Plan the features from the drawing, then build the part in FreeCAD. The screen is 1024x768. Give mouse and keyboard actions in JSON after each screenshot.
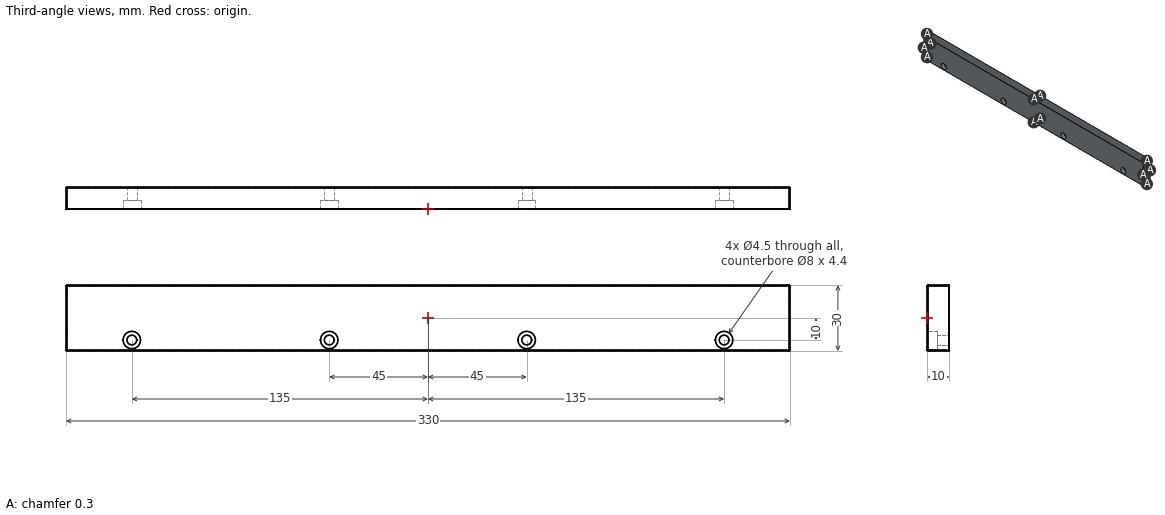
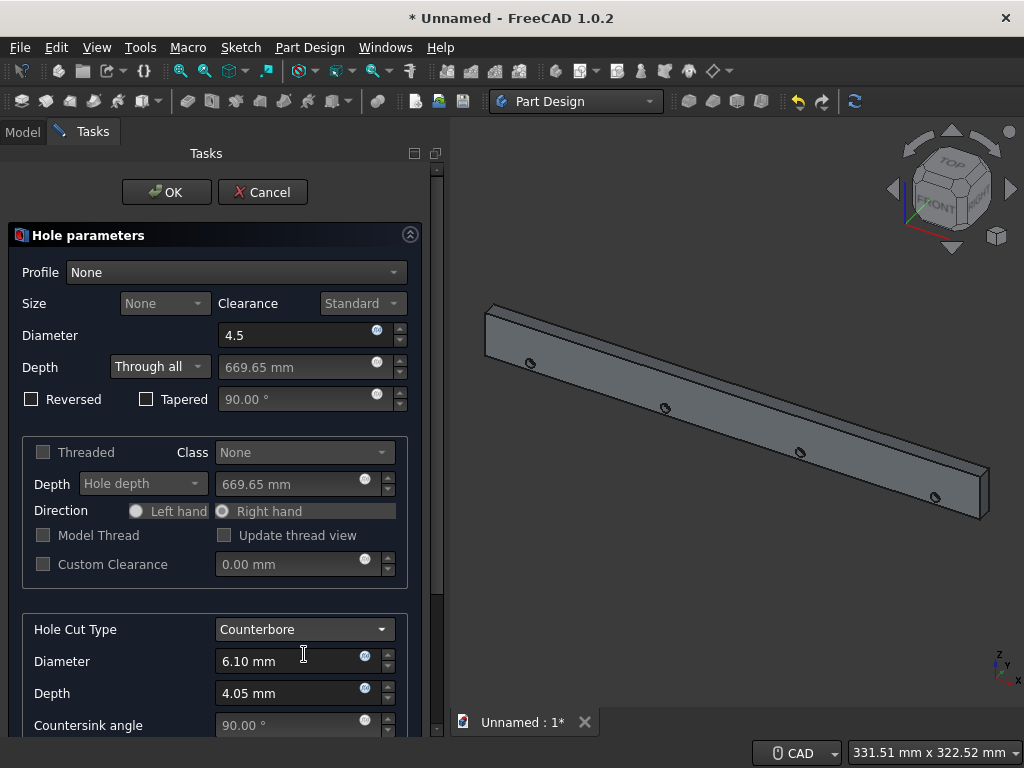
{"action": "triple_click", "coordinate": [298, 661]}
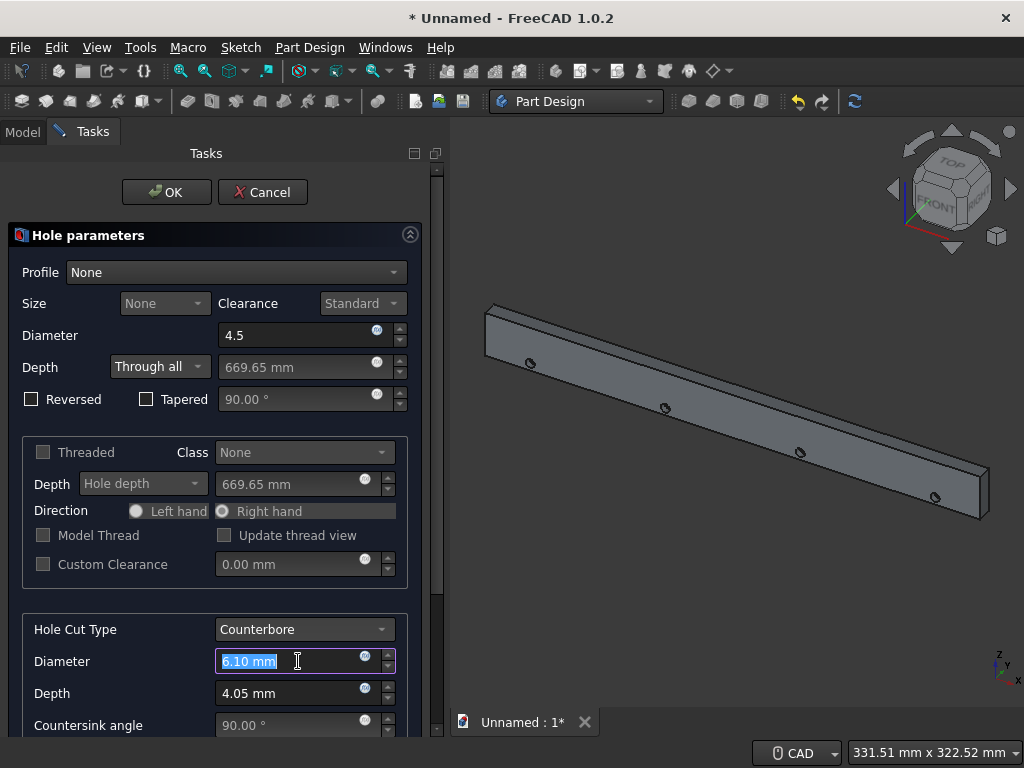
{"action": "type", "text": "8"}
{"action": "key", "text": "Tab"}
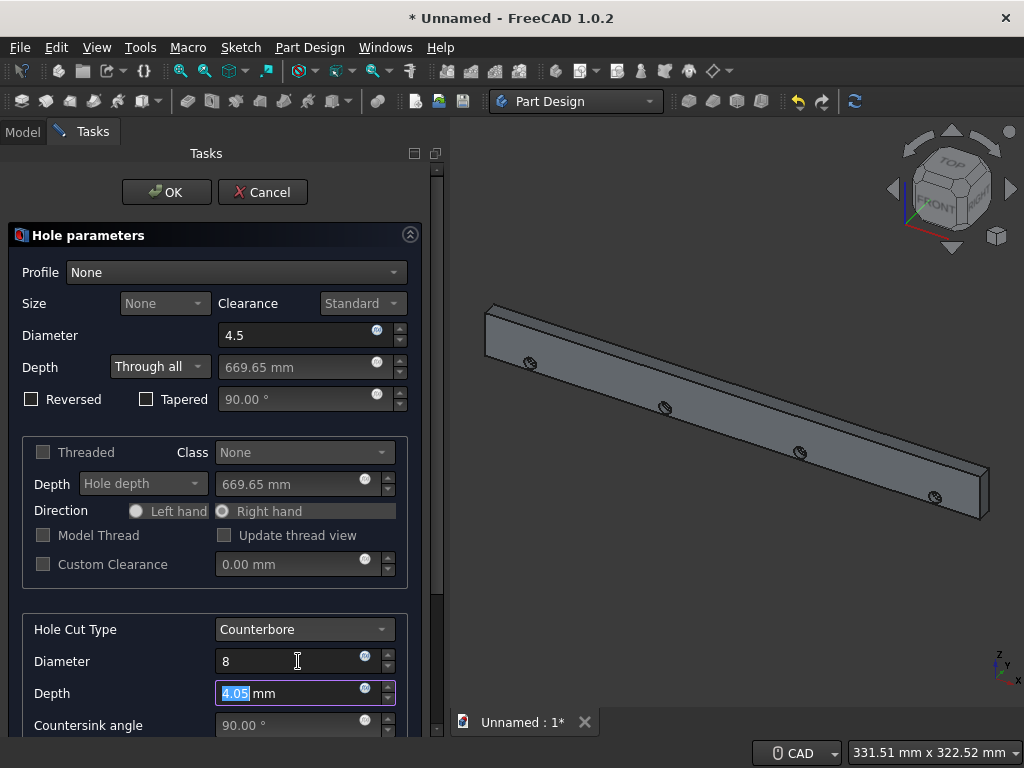
{"action": "type", "text": "4.4"}
{"action": "key", "text": "Tab"}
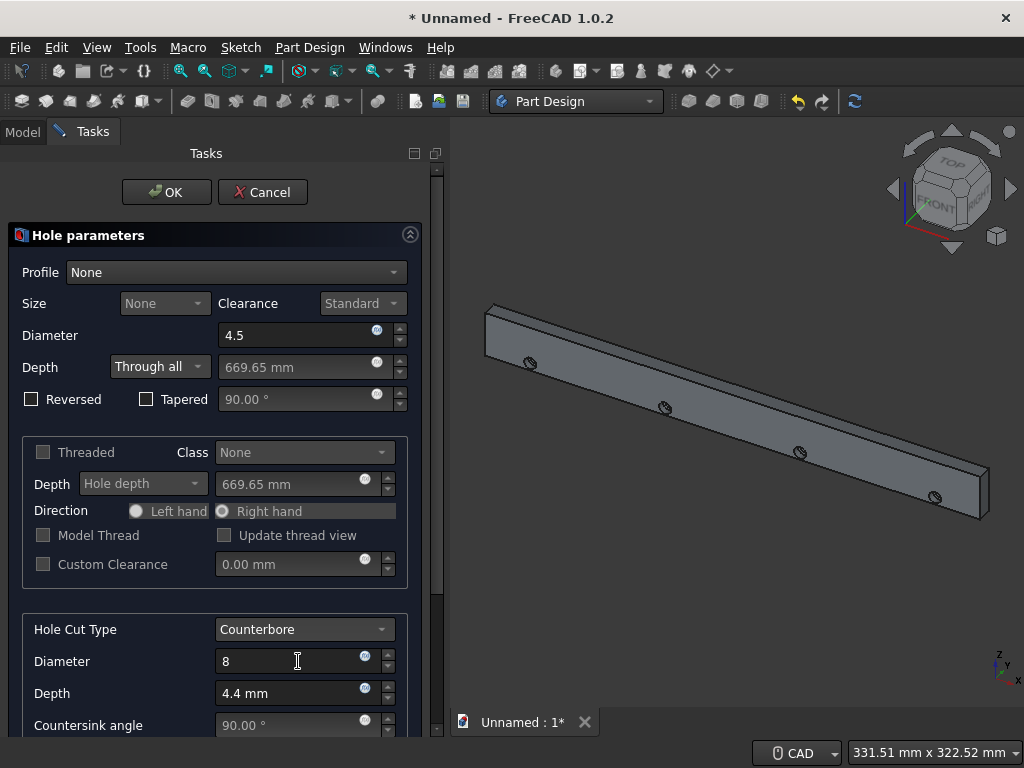
{"action": "left_click", "coordinate": [167, 192]}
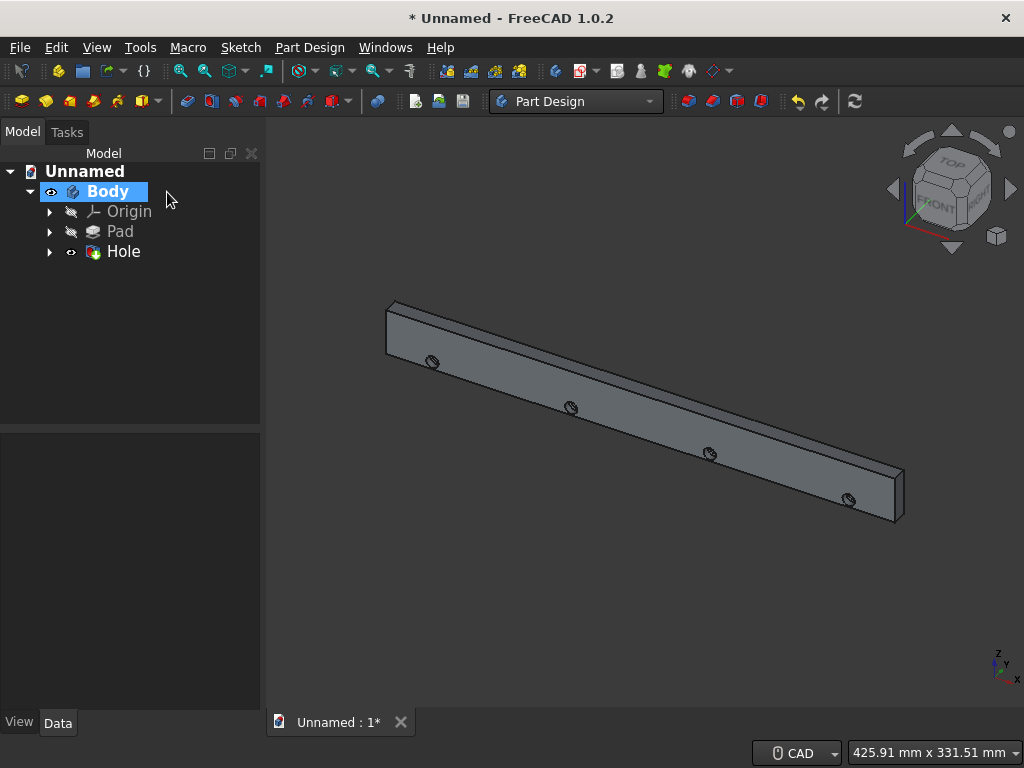
{"action": "left_click", "coordinate": [895, 500]}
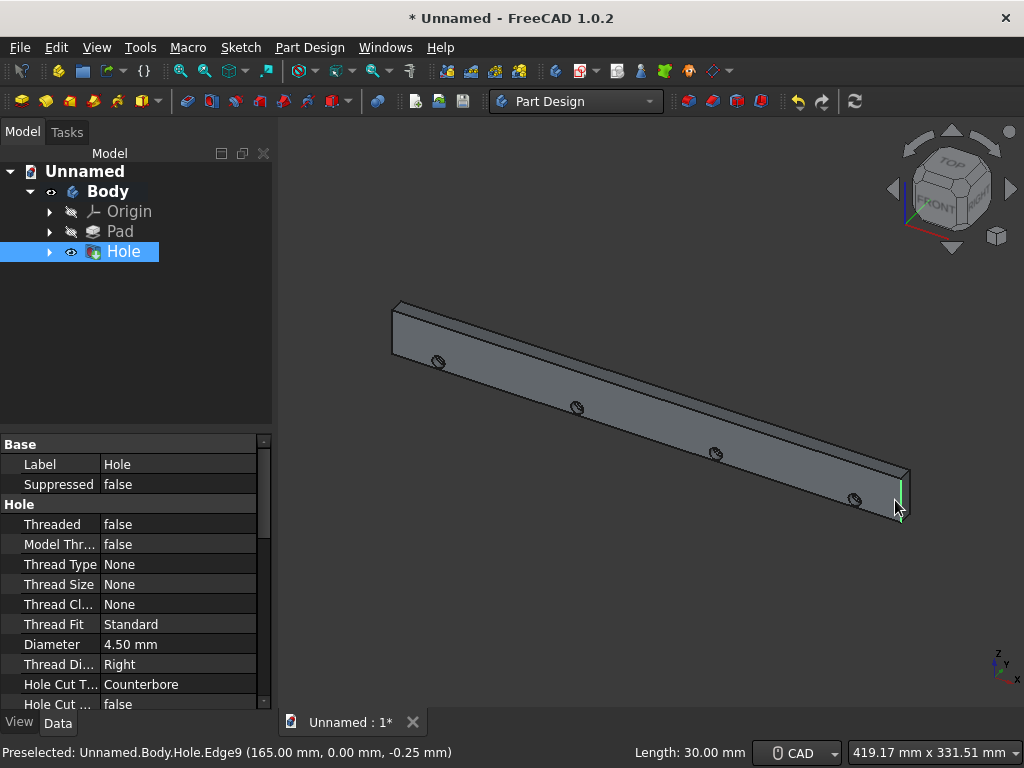
{"action": "key", "text": "0"}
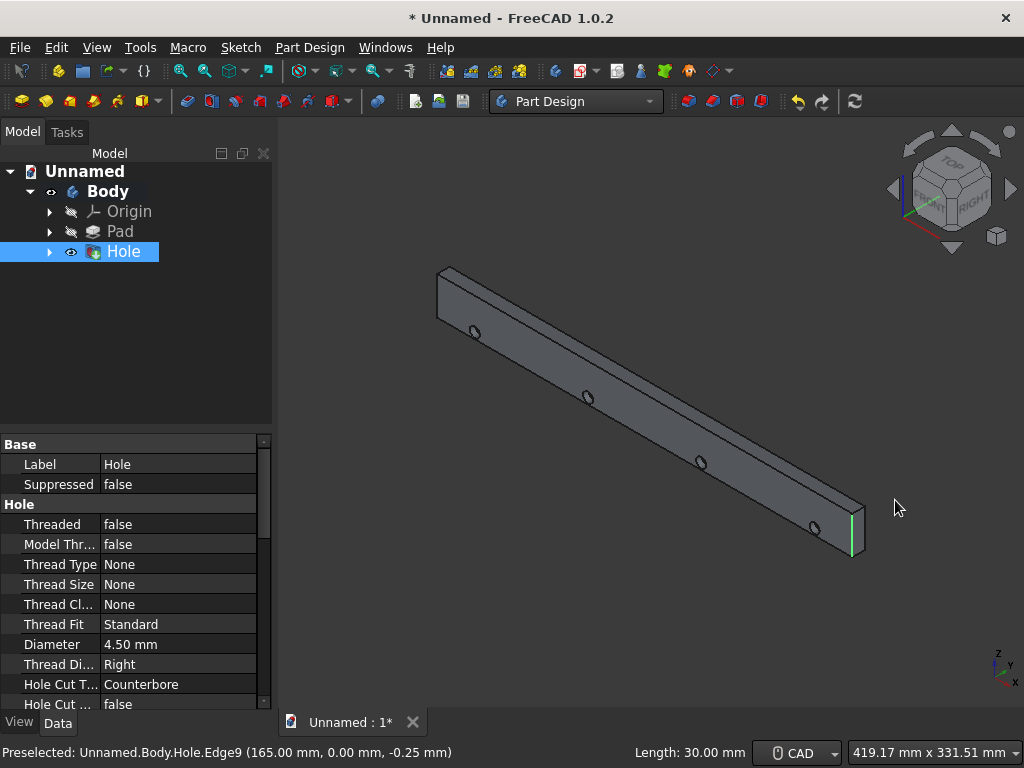
{"action": "key", "text": "2"}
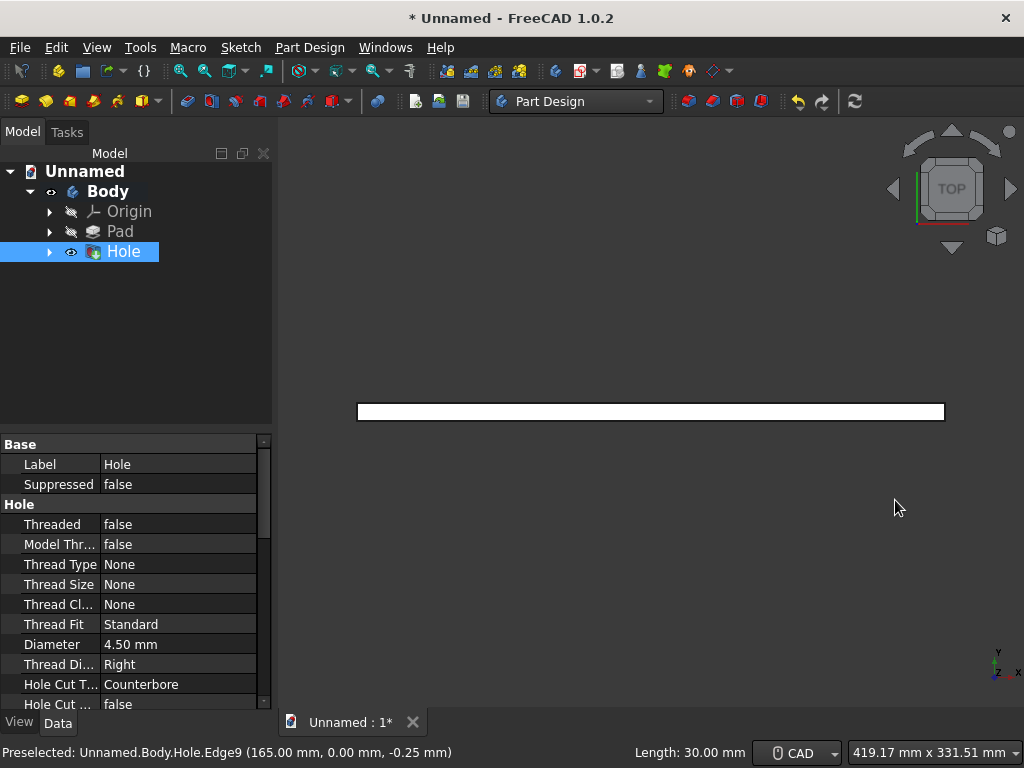
{"action": "left_click", "coordinate": [903, 411], "text": "ctrl"}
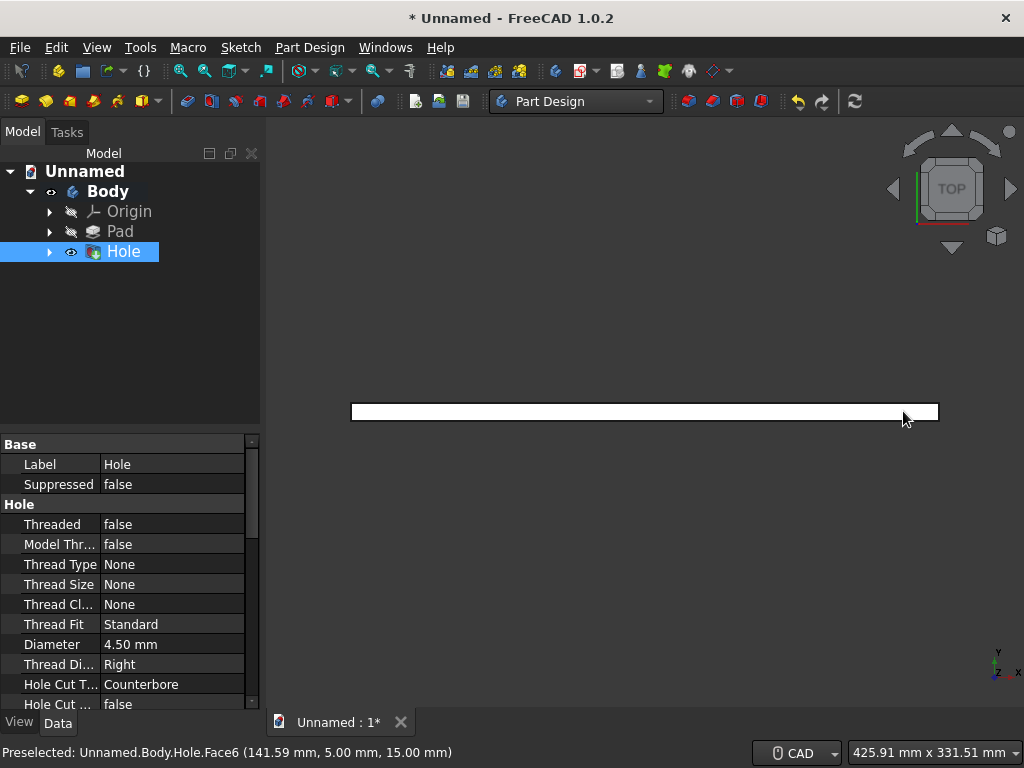
{"action": "key", "text": "1"}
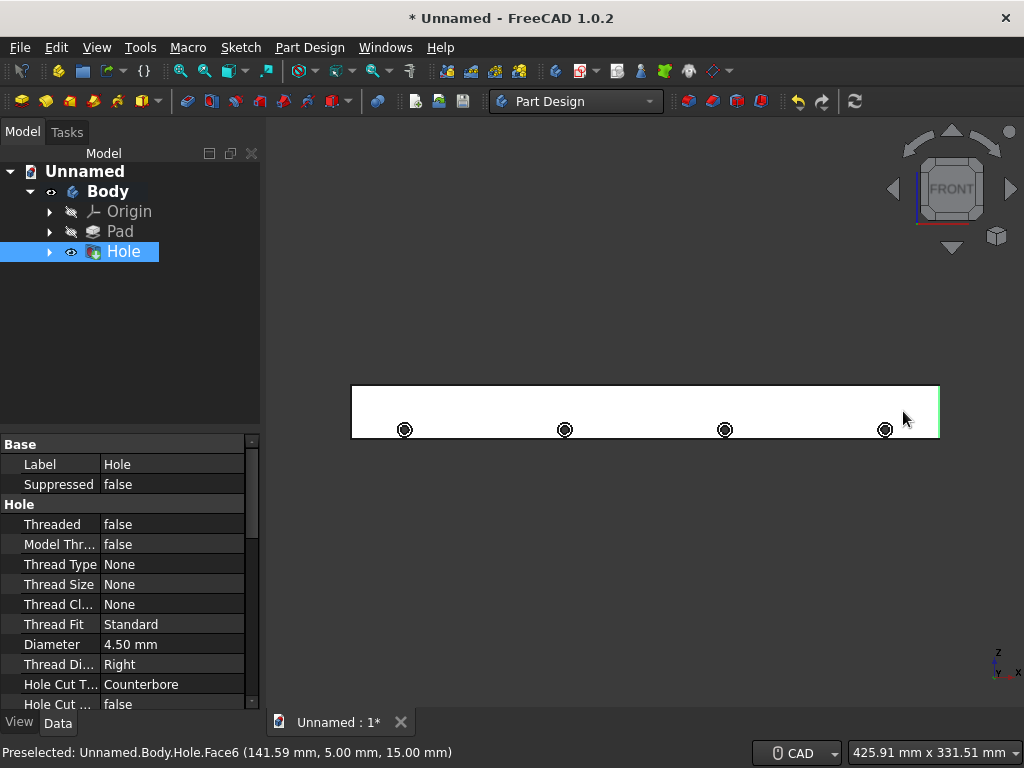
{"action": "left_click", "coordinate": [351, 411], "text": "ctrl"}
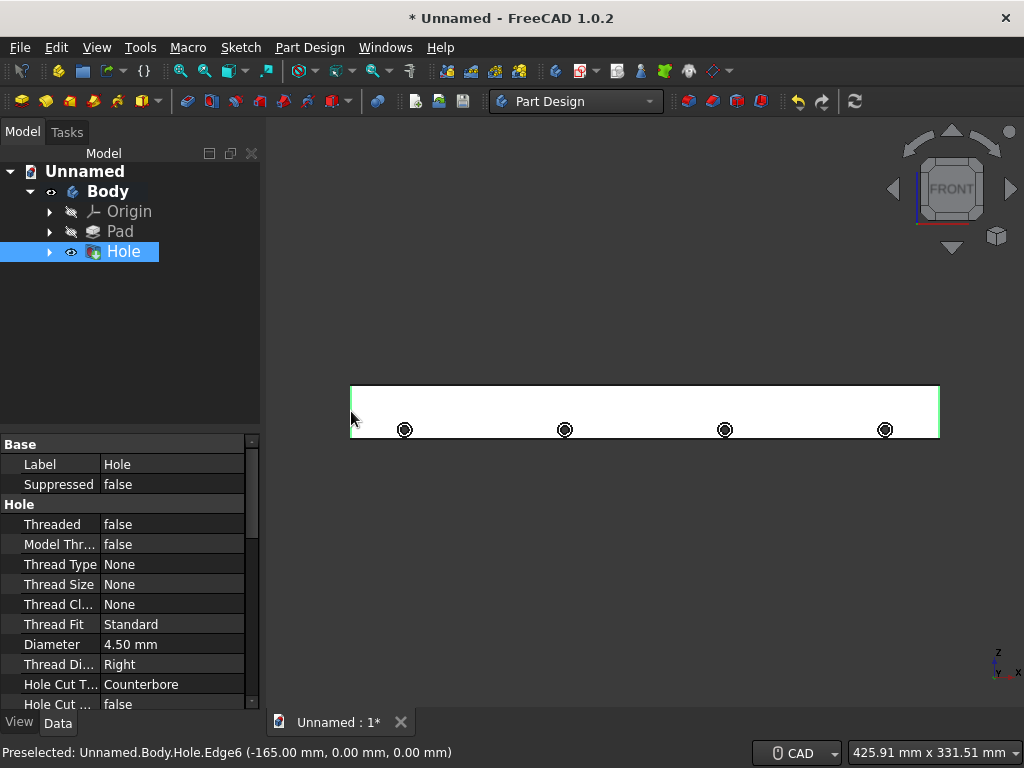
{"action": "key", "text": "3"}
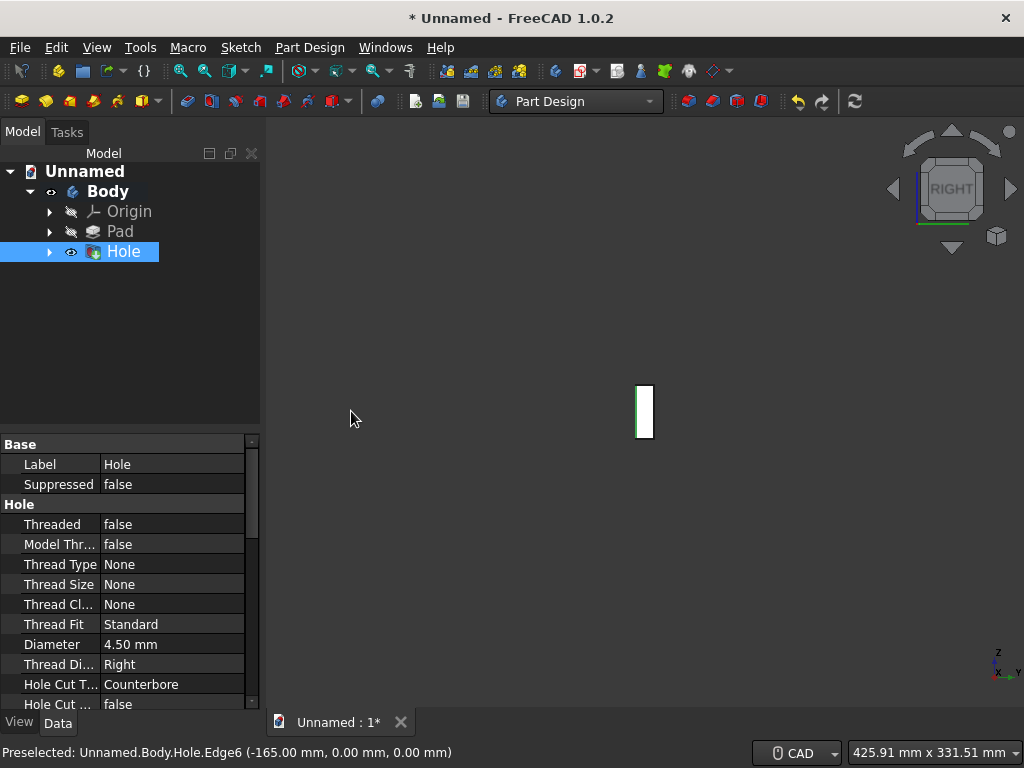
{"action": "left_click", "coordinate": [182, 72]}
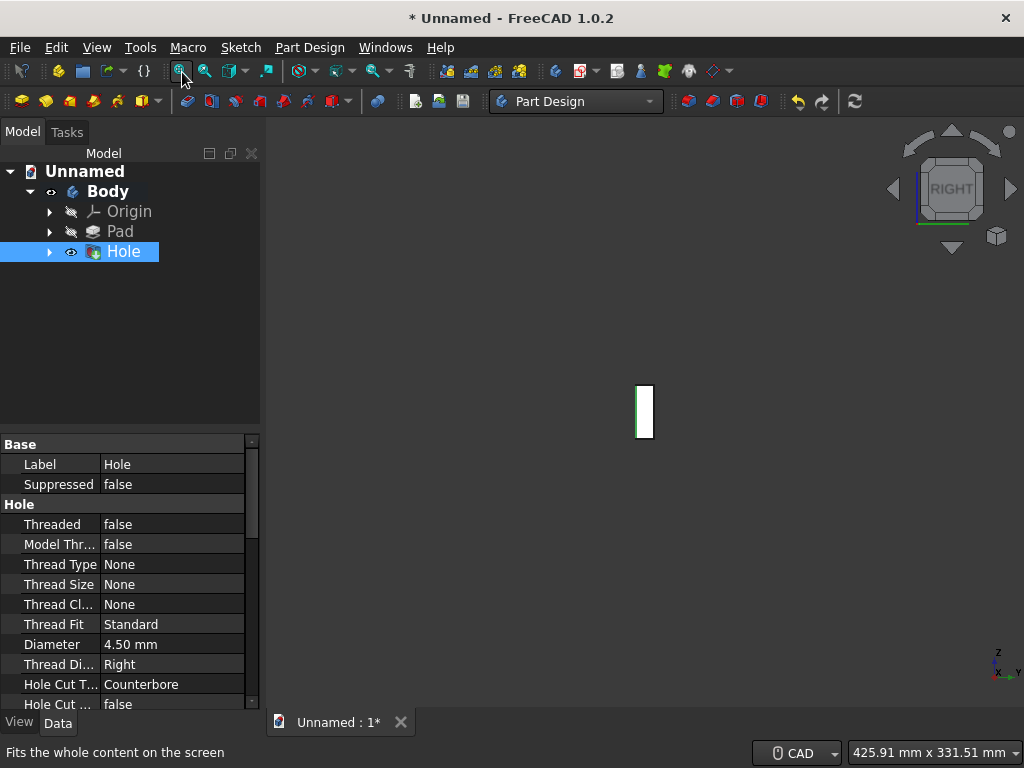
{"action": "left_click", "coordinate": [654, 411], "text": "ctrl"}